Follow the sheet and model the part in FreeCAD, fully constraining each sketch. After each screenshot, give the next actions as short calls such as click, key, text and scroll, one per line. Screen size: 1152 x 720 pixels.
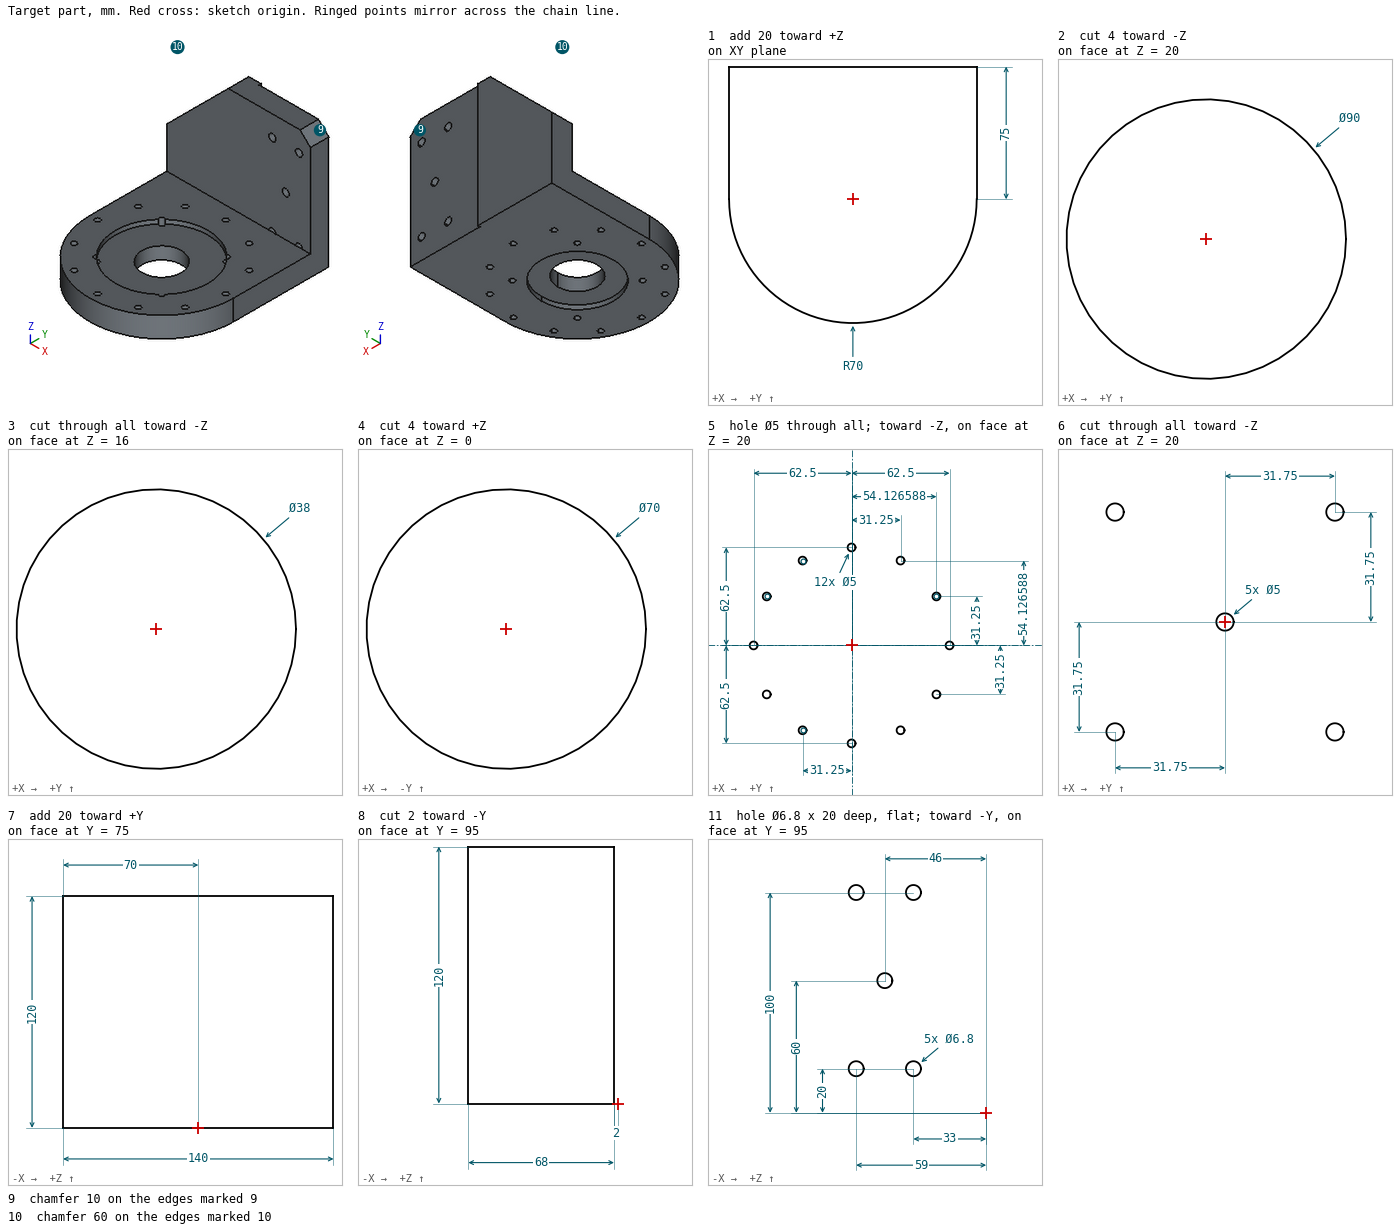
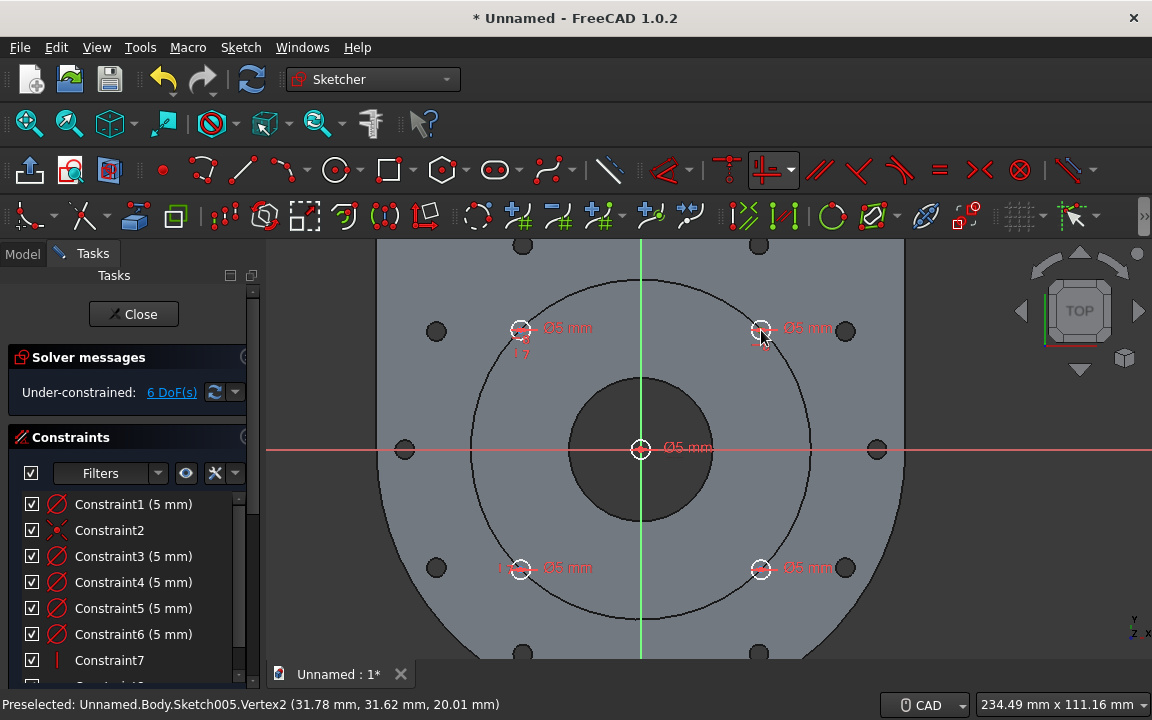
click(761, 570)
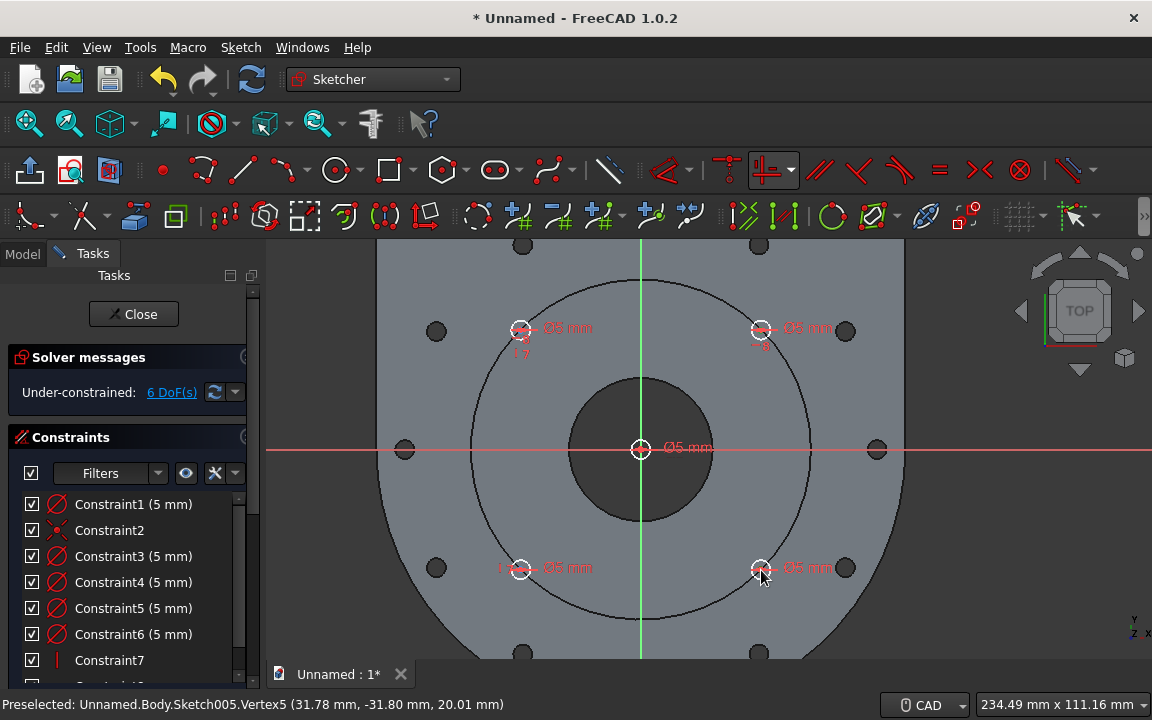
key(v)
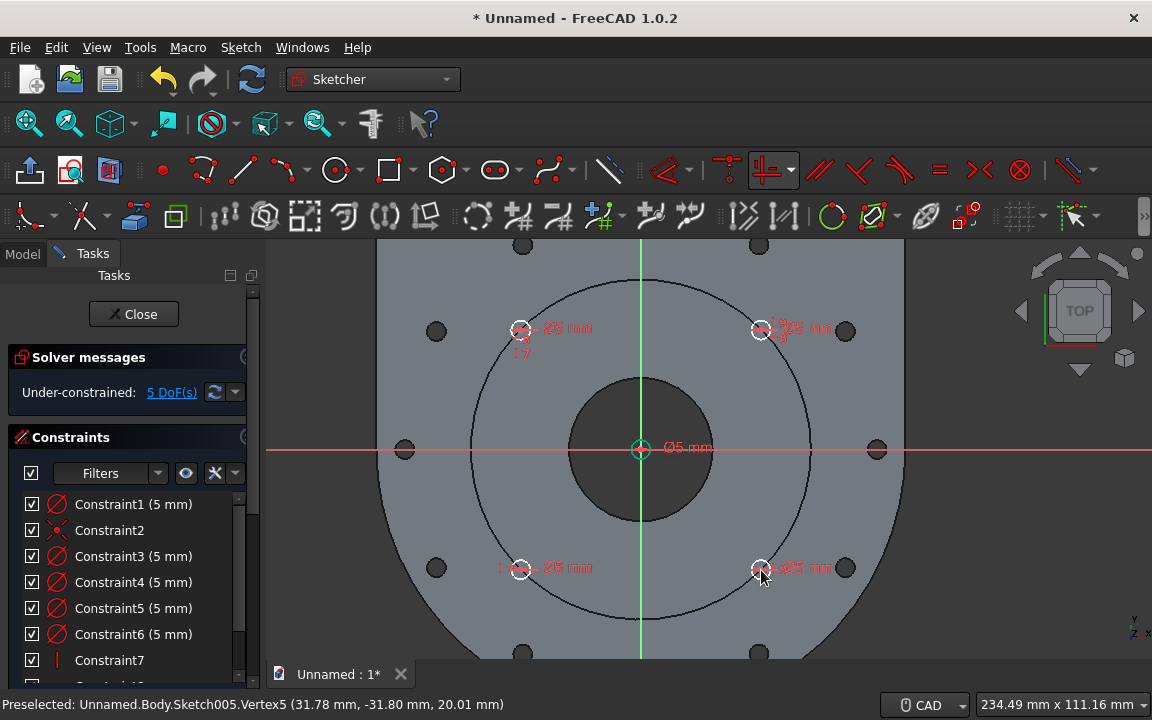
click(521, 570)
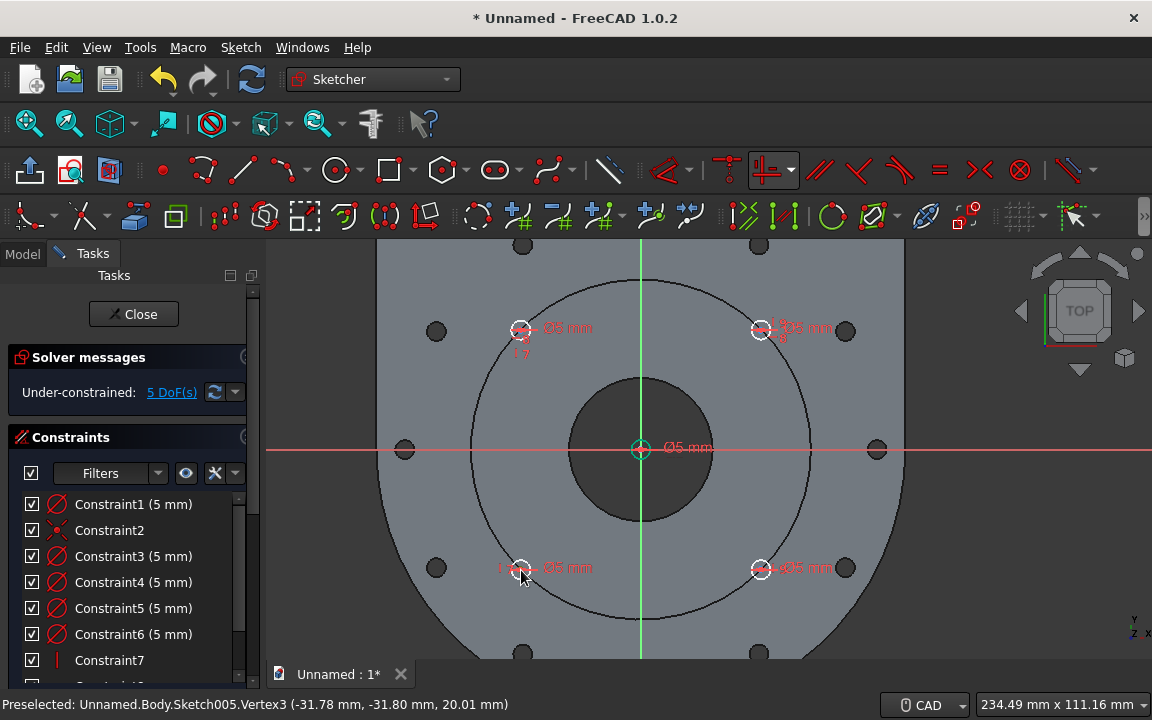
click(761, 570)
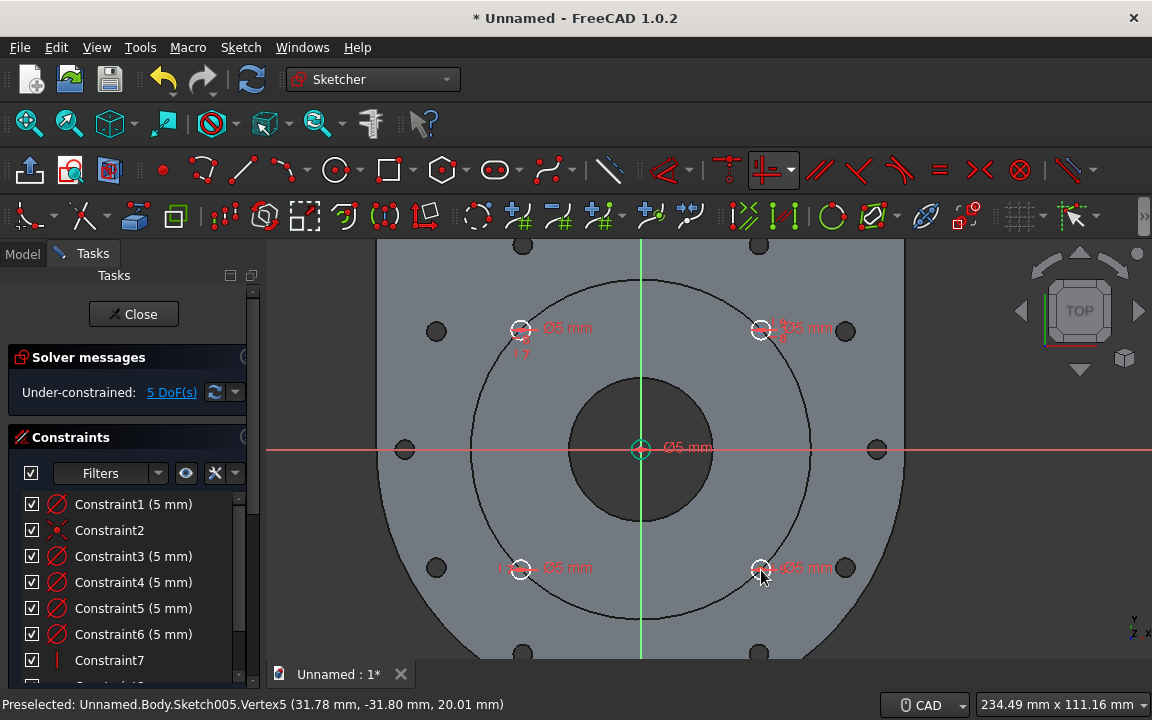
key(h)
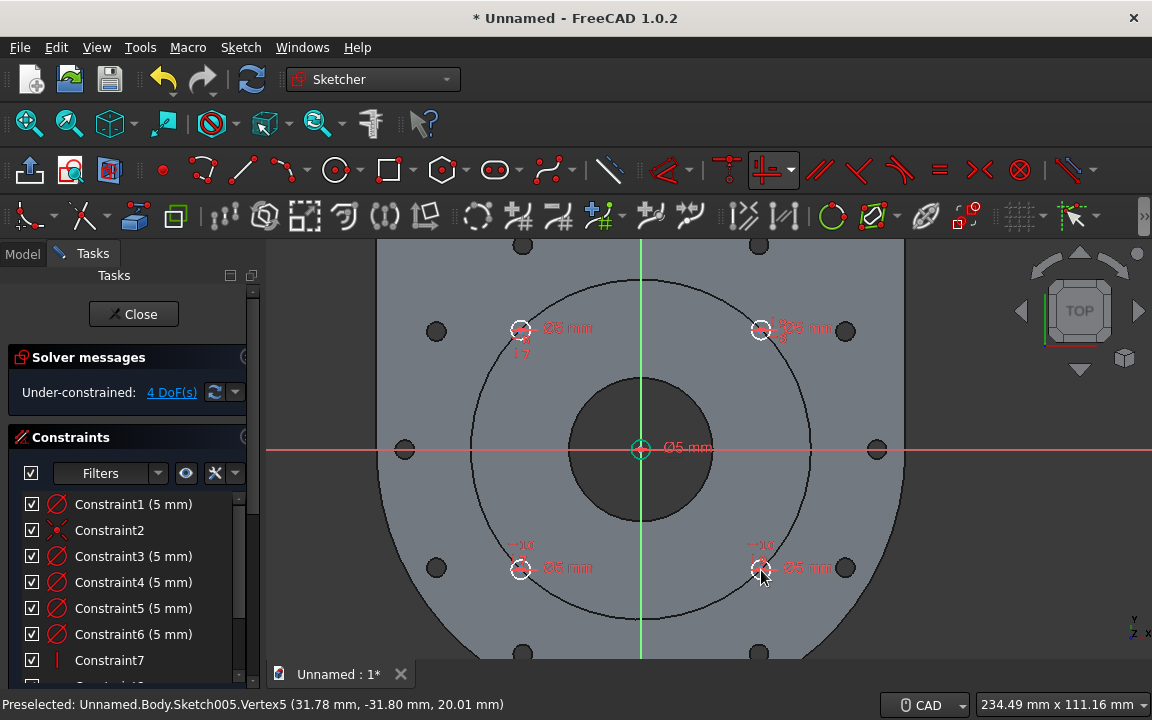
key(d)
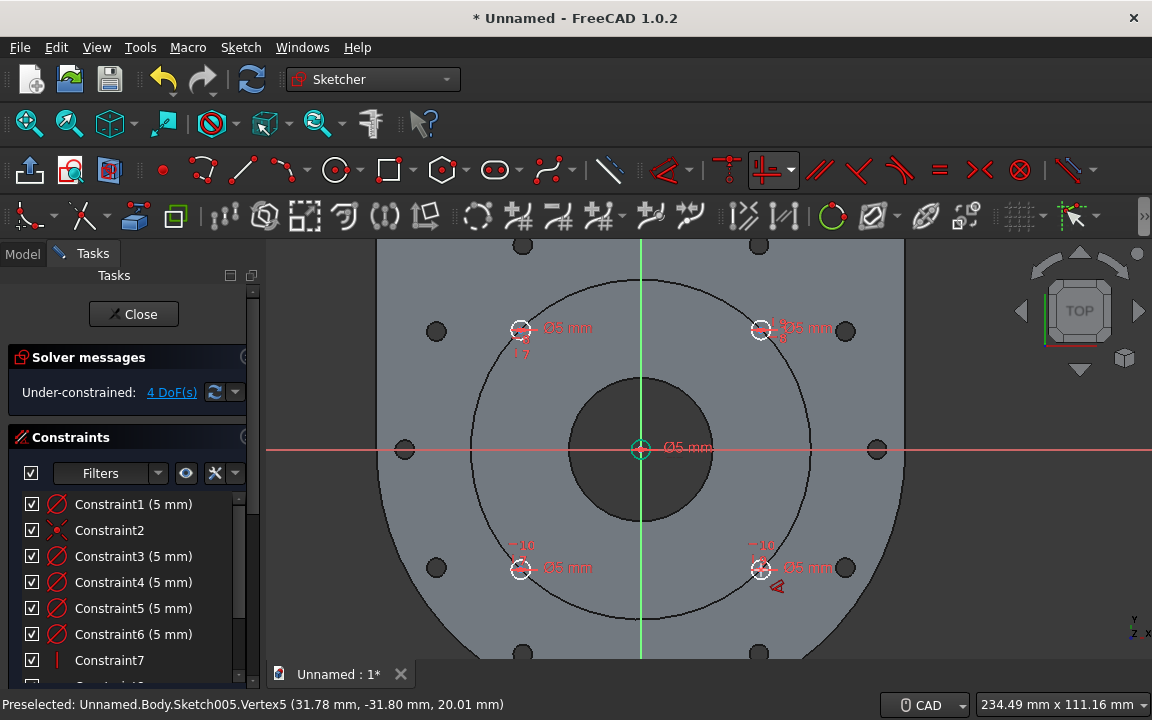
click(761, 330)
click(701, 296)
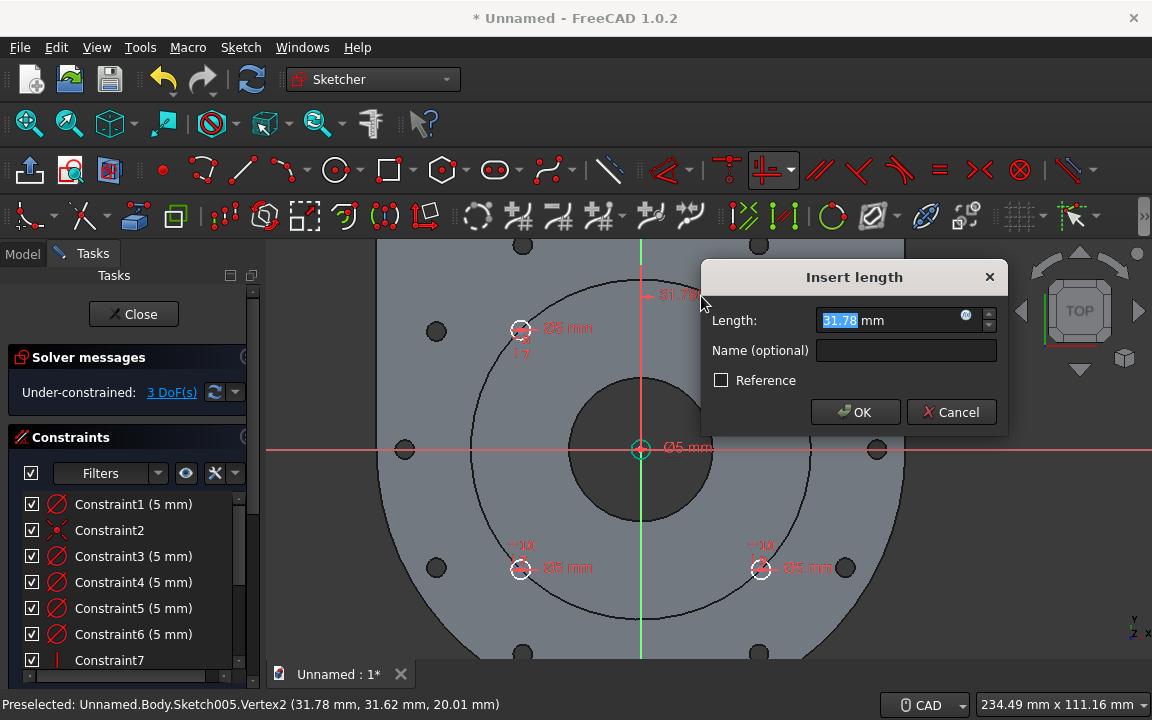
text(31.75)
key(Return)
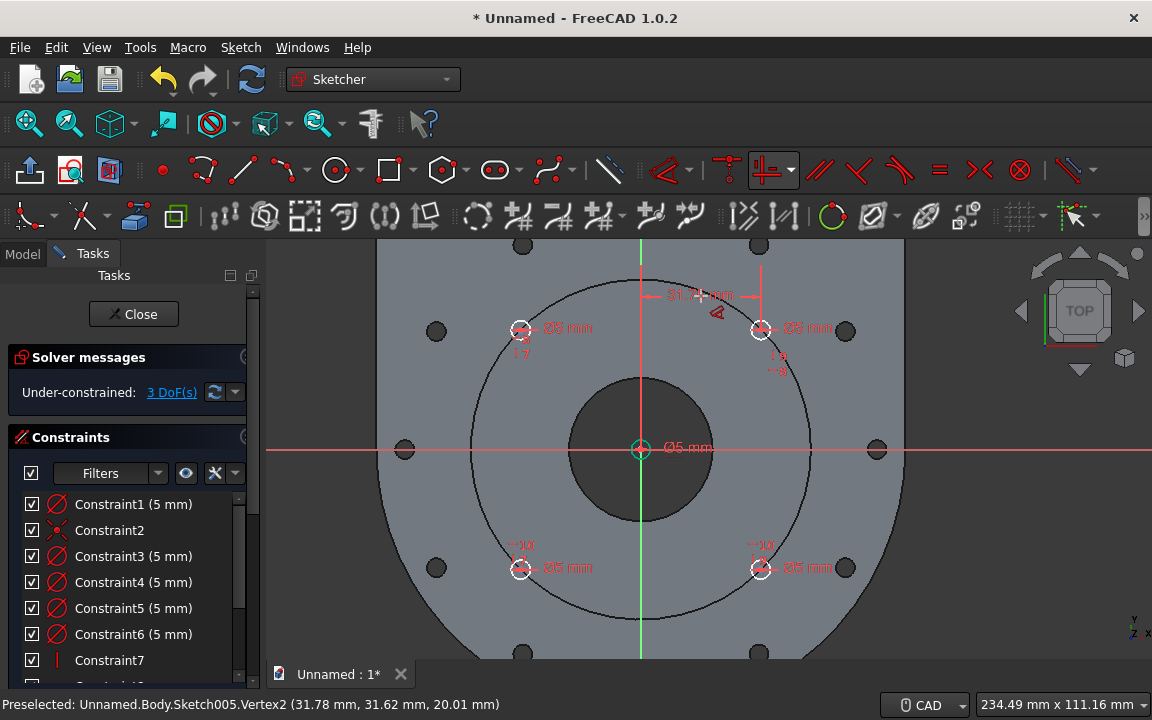
click(761, 330)
click(795, 390)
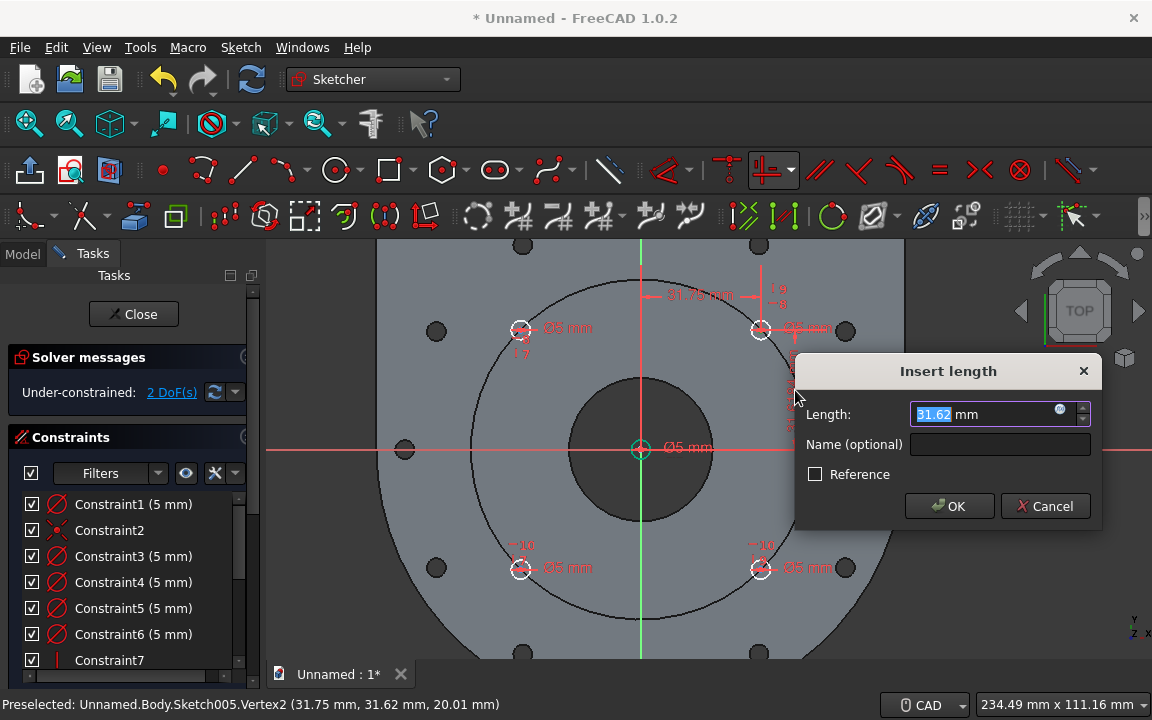
text(31.75)
key(Return)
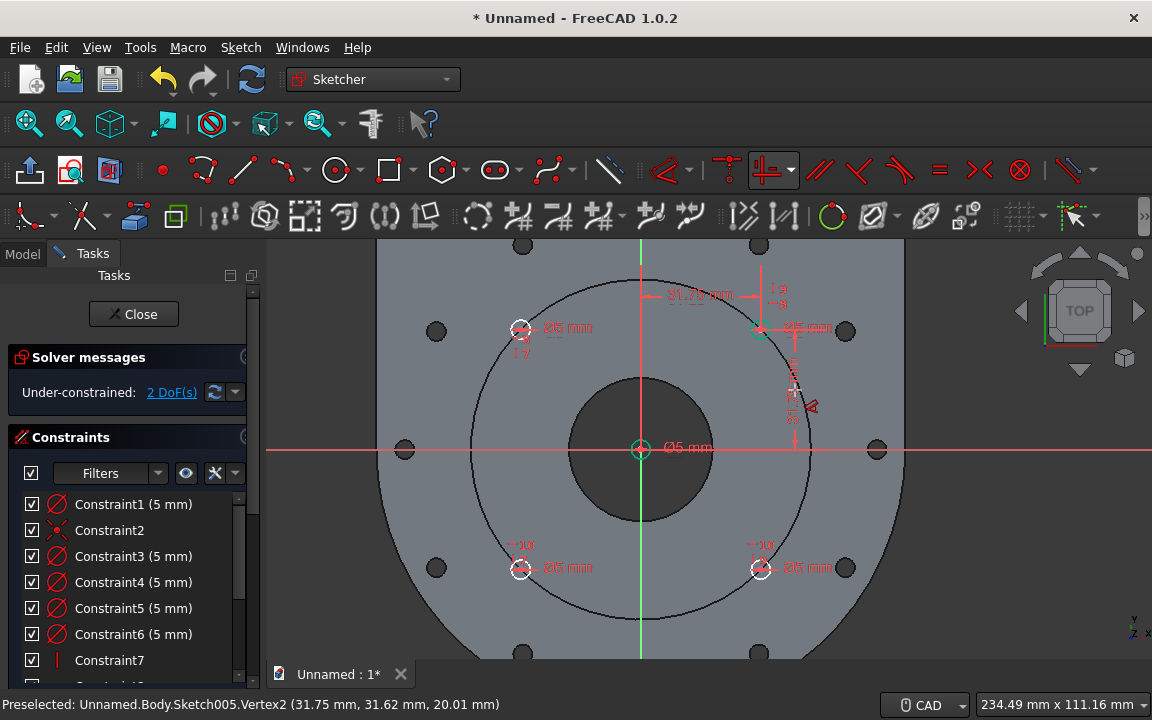
click(521, 570)
click(581, 604)